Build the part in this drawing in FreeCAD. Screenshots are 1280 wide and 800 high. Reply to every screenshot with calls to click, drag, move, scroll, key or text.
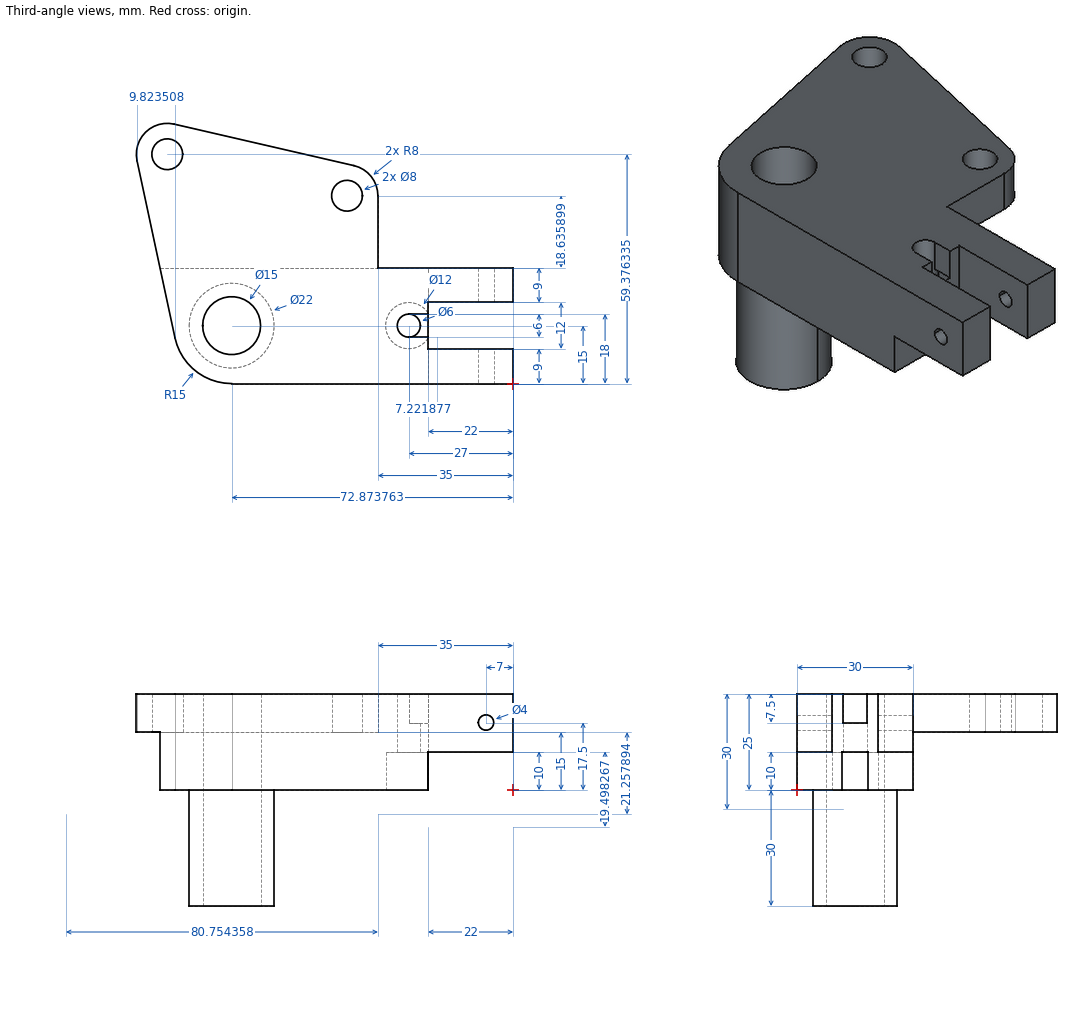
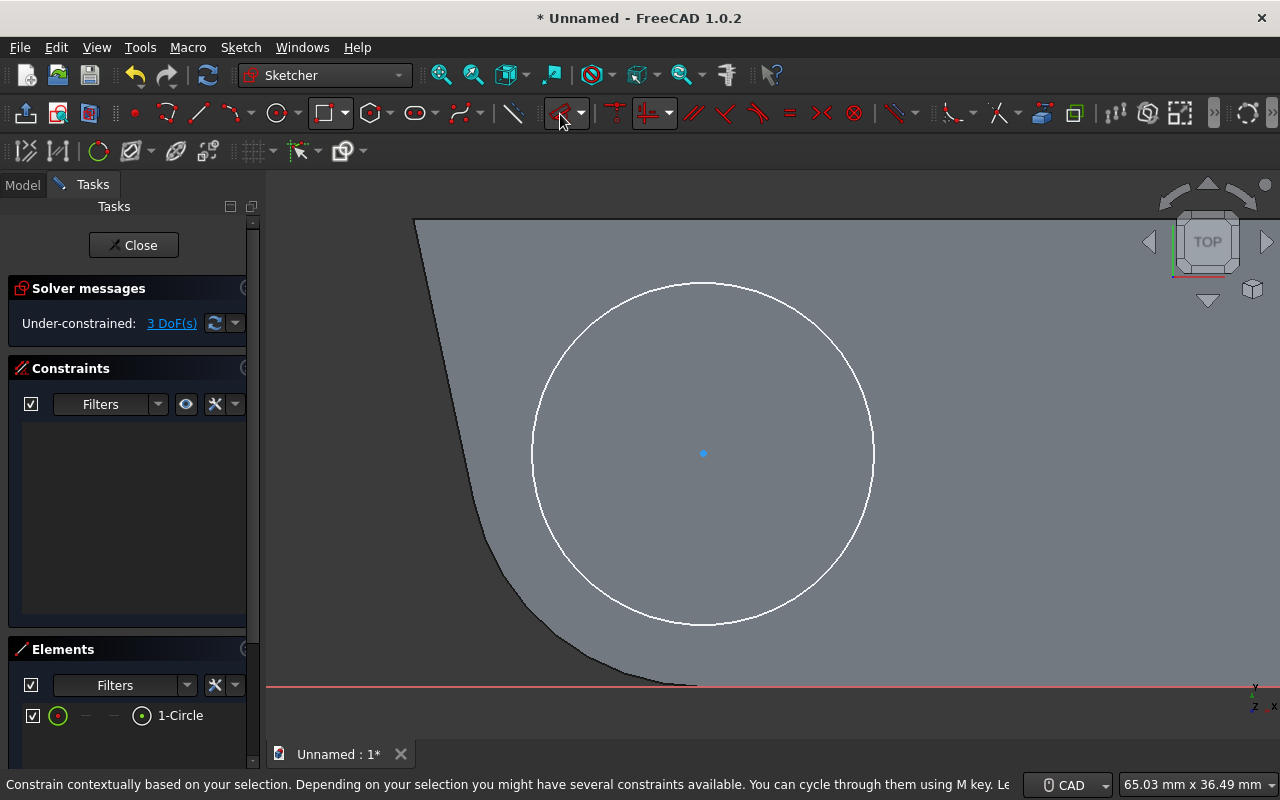
click(824, 333)
click(847, 310)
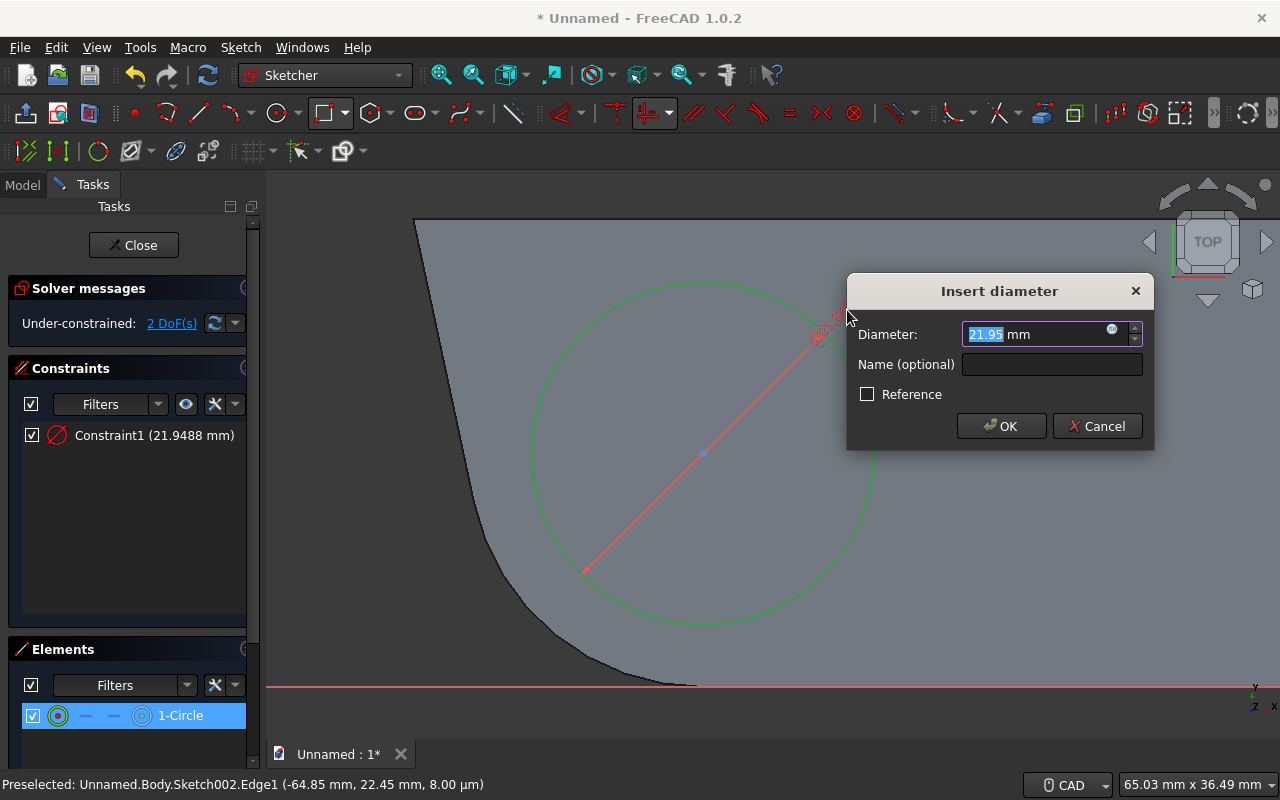
text(22)
key(Return)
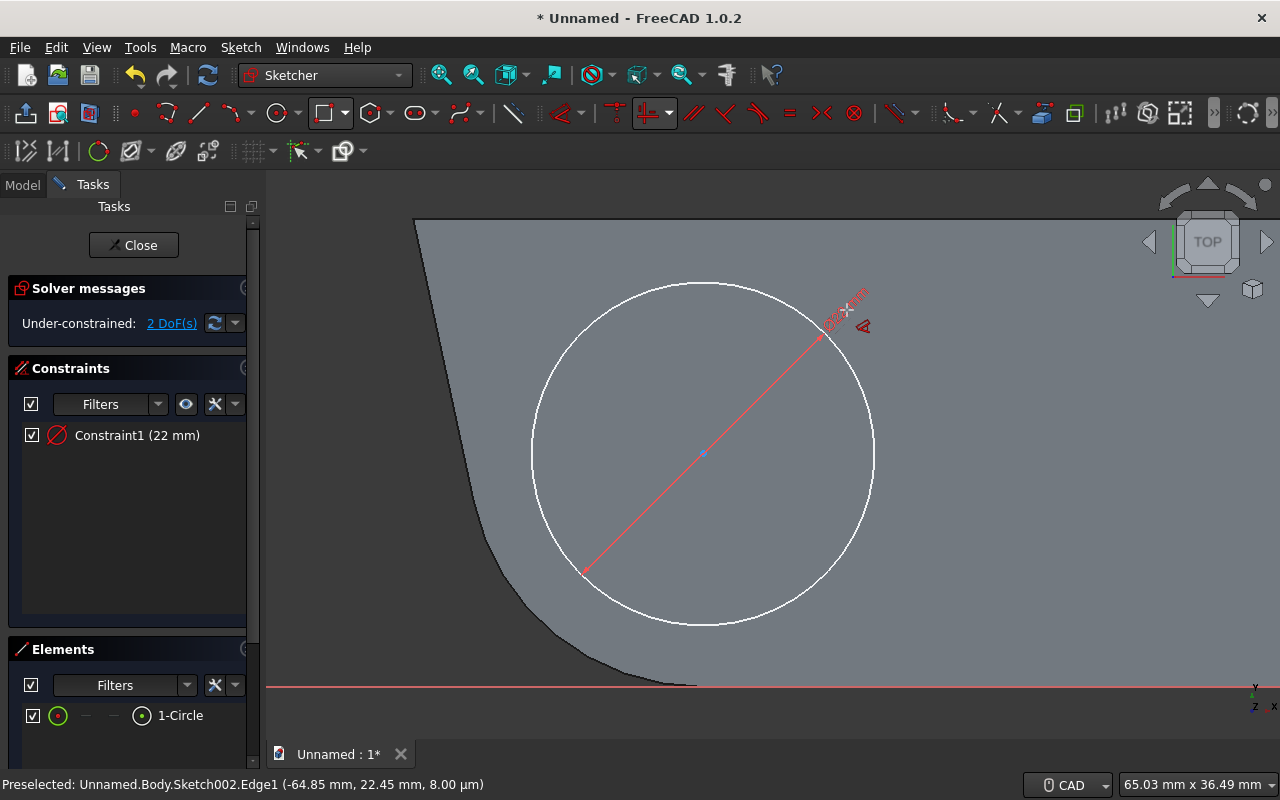
click(703, 454)
click(669, 570)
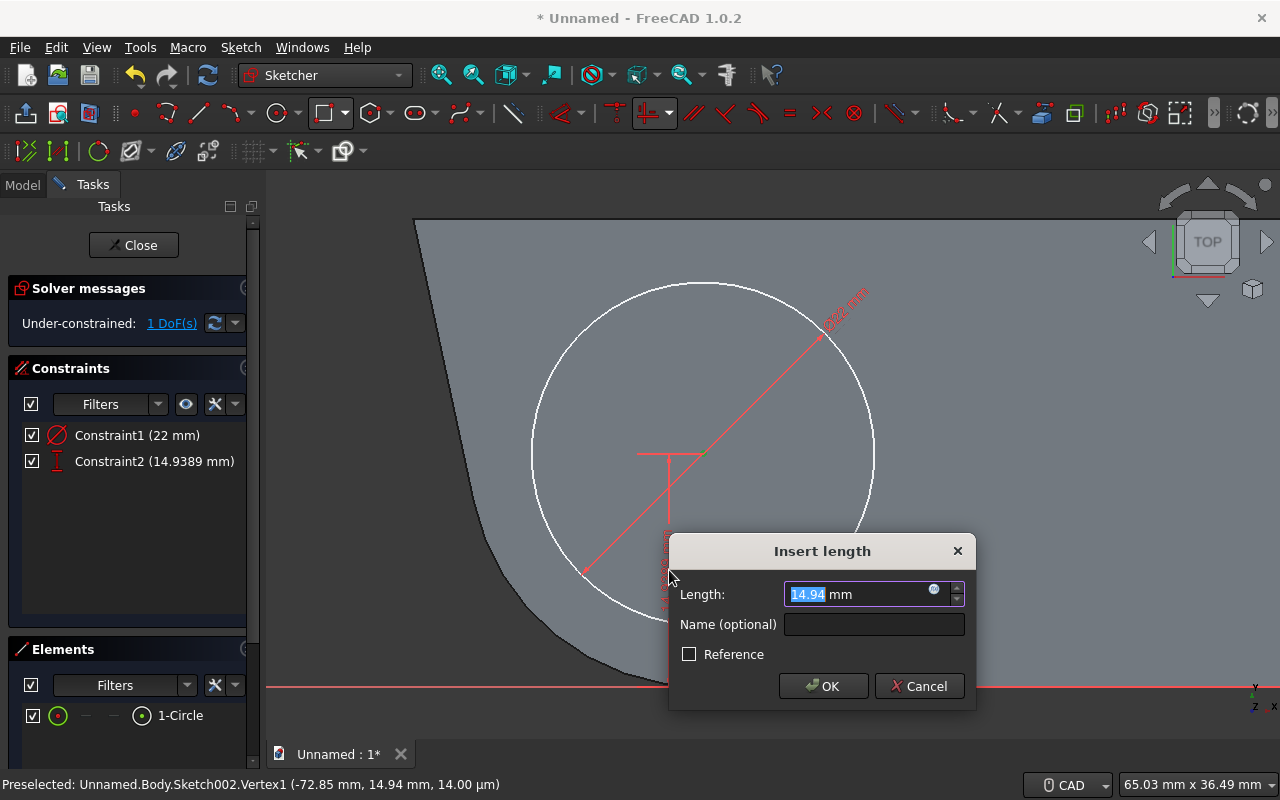
text(15)
key(Return)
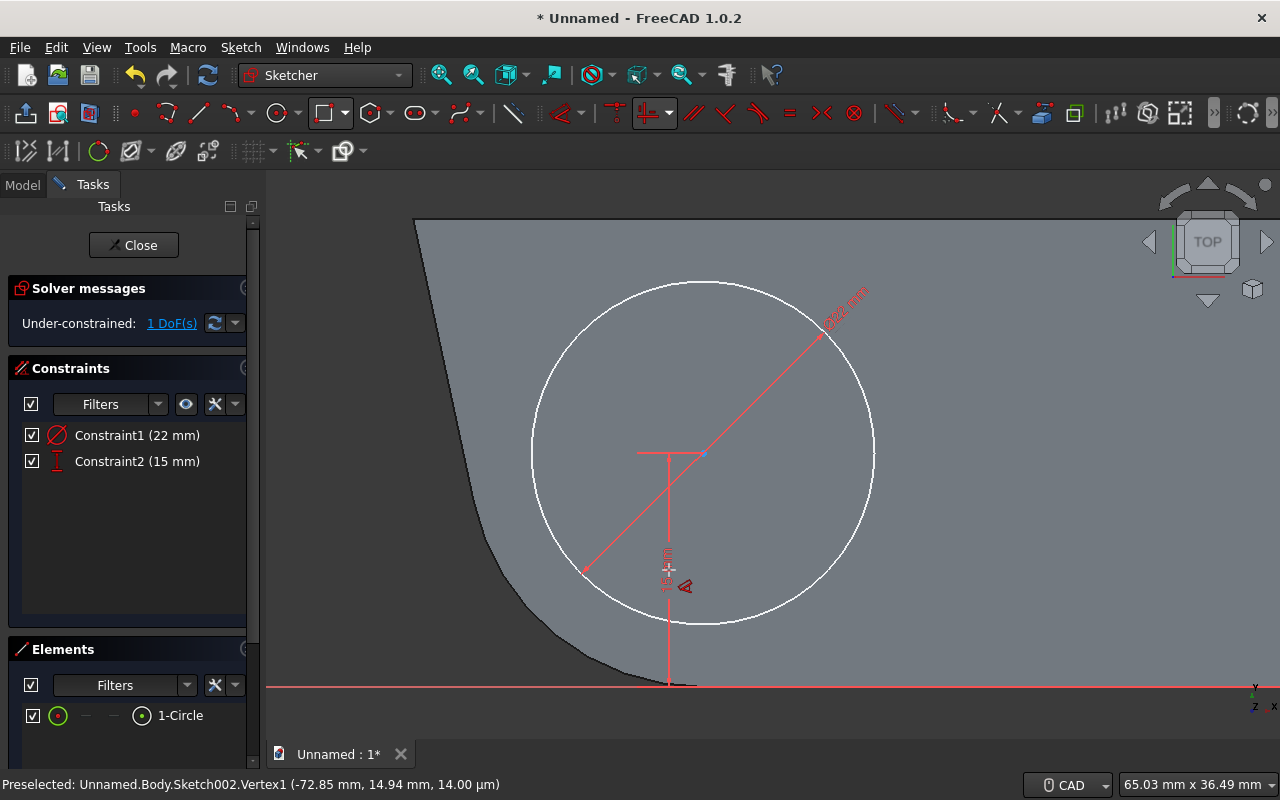
click(703, 453)
click(909, 419)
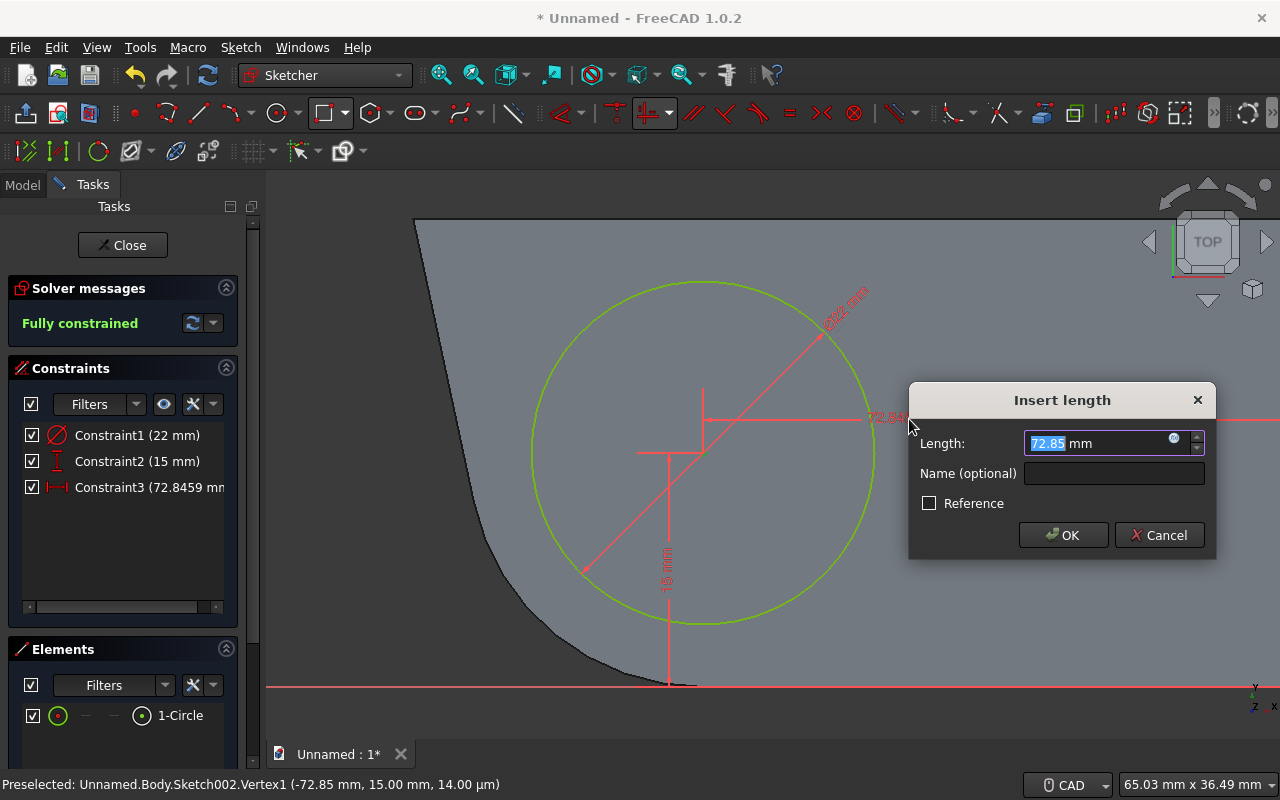
text(72.873763)
key(Return)
key(Escape)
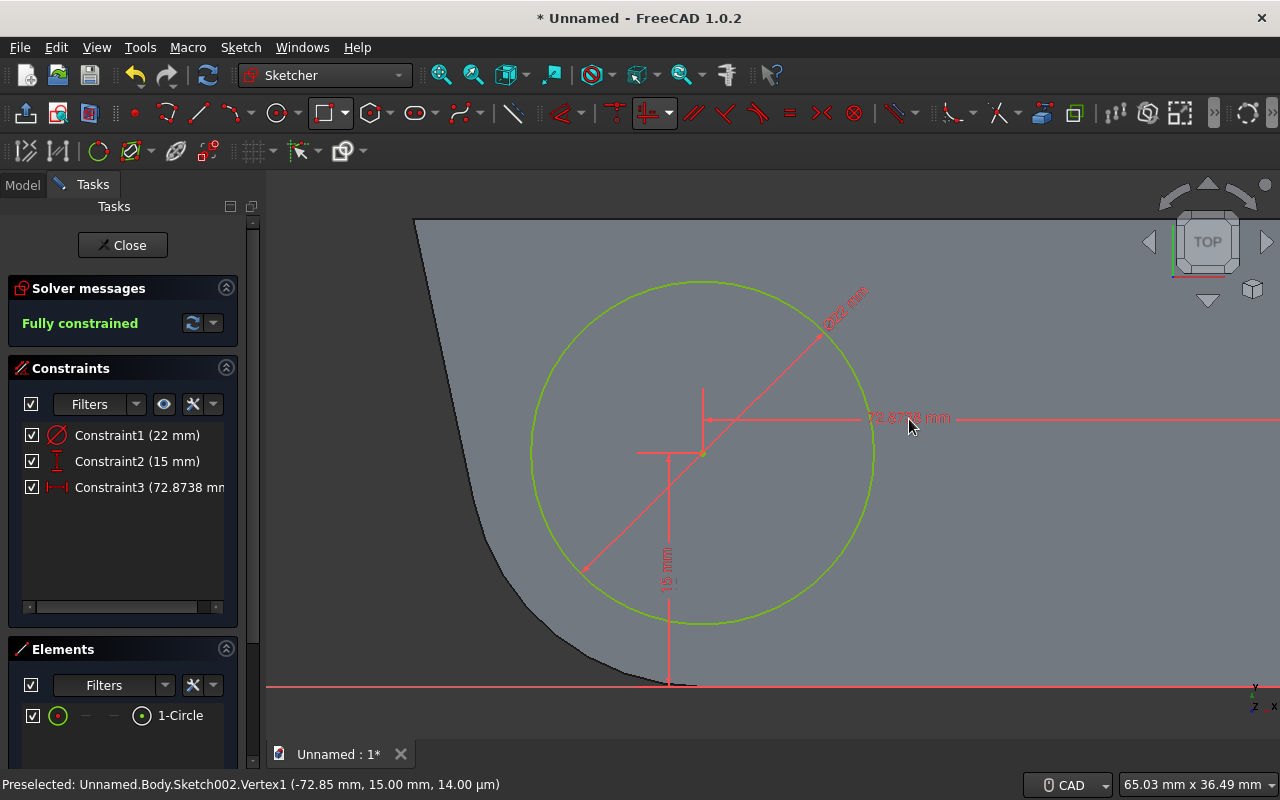
click(123, 245)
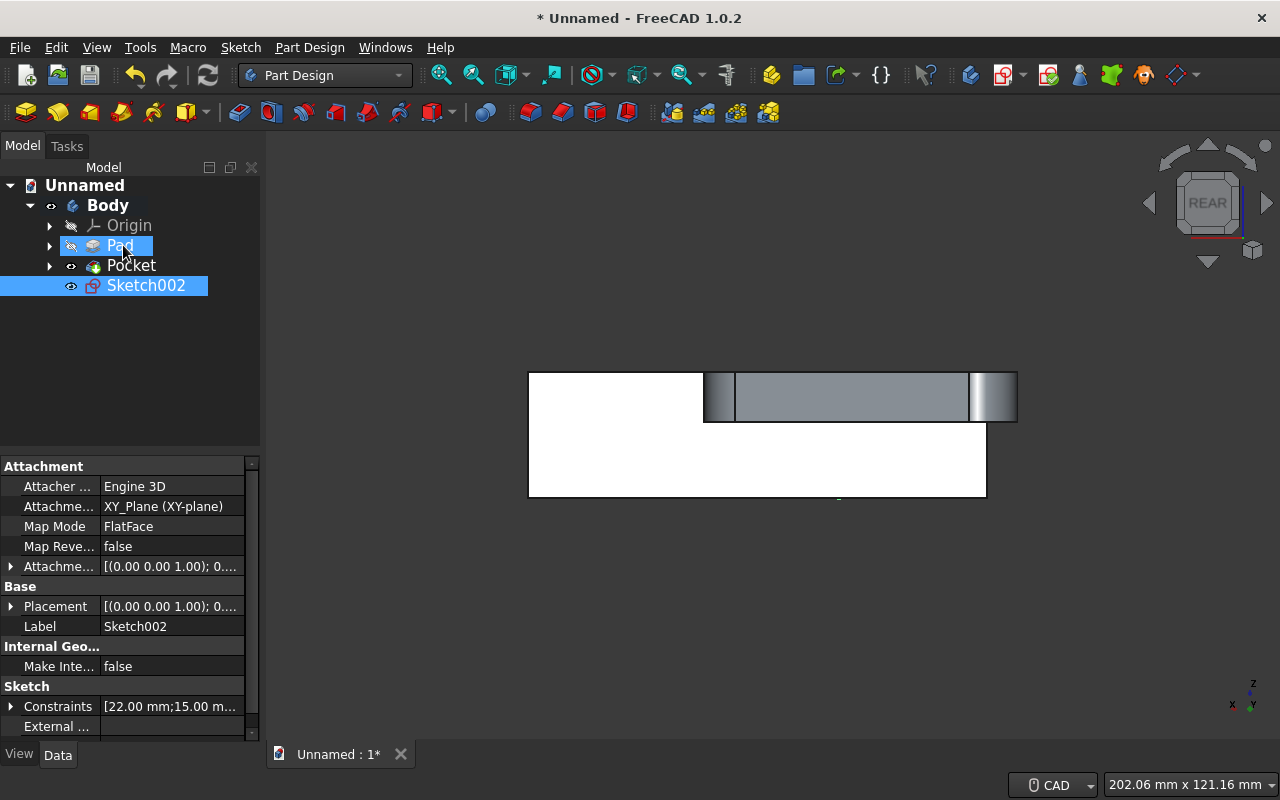
click(26, 112)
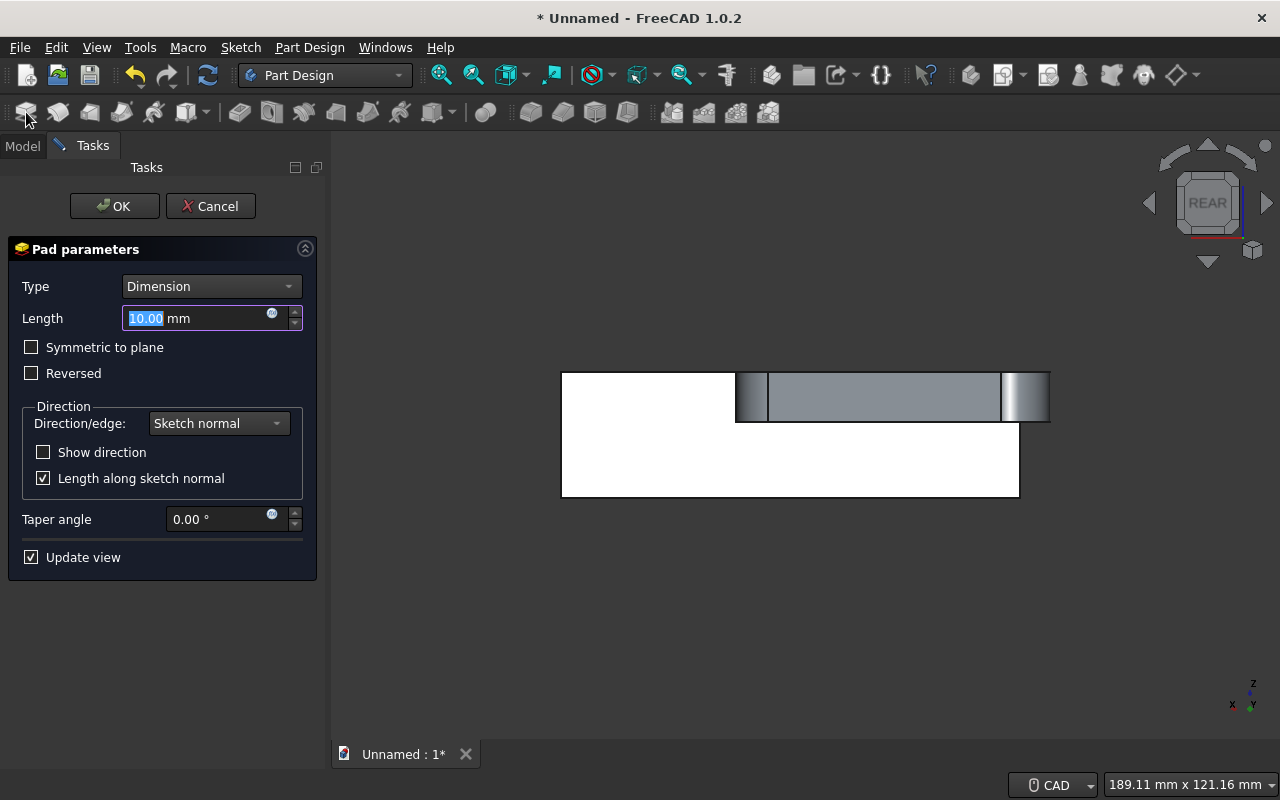
text(30)
key(Tab)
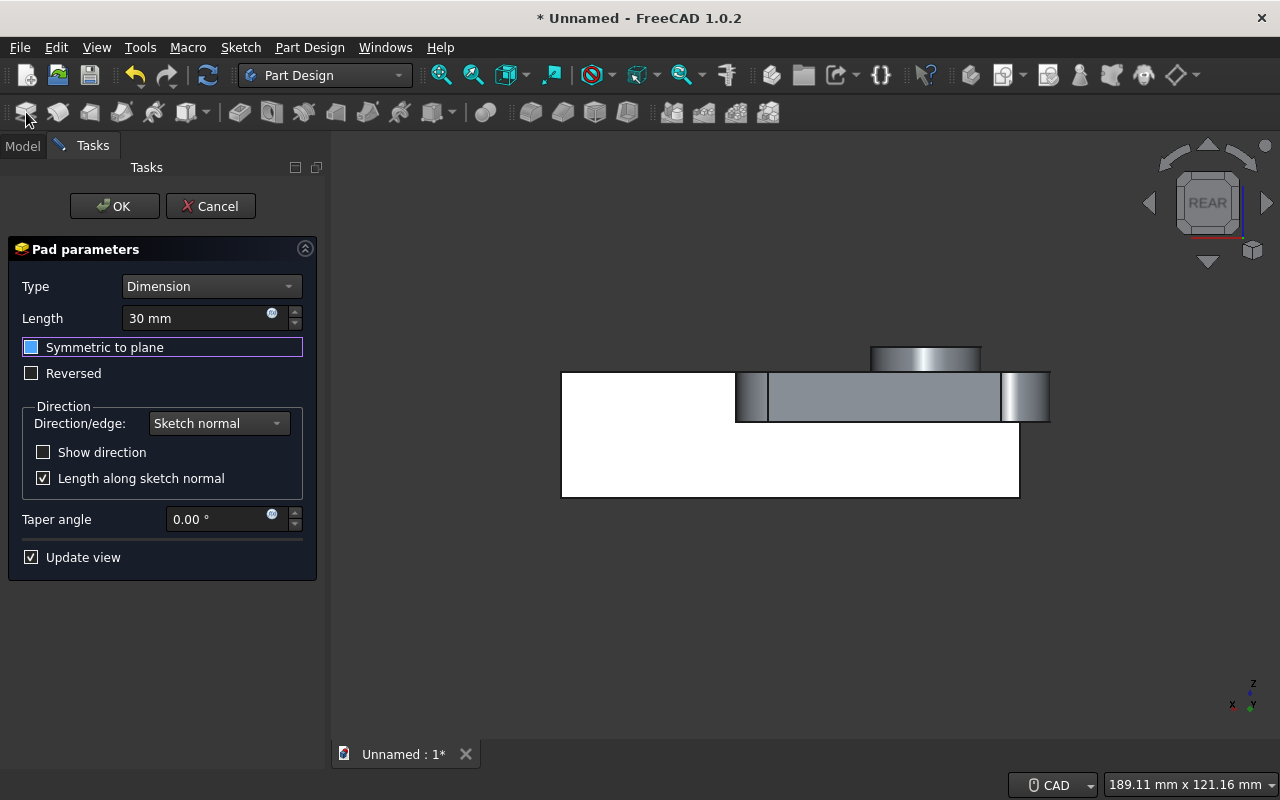
click(30, 373)